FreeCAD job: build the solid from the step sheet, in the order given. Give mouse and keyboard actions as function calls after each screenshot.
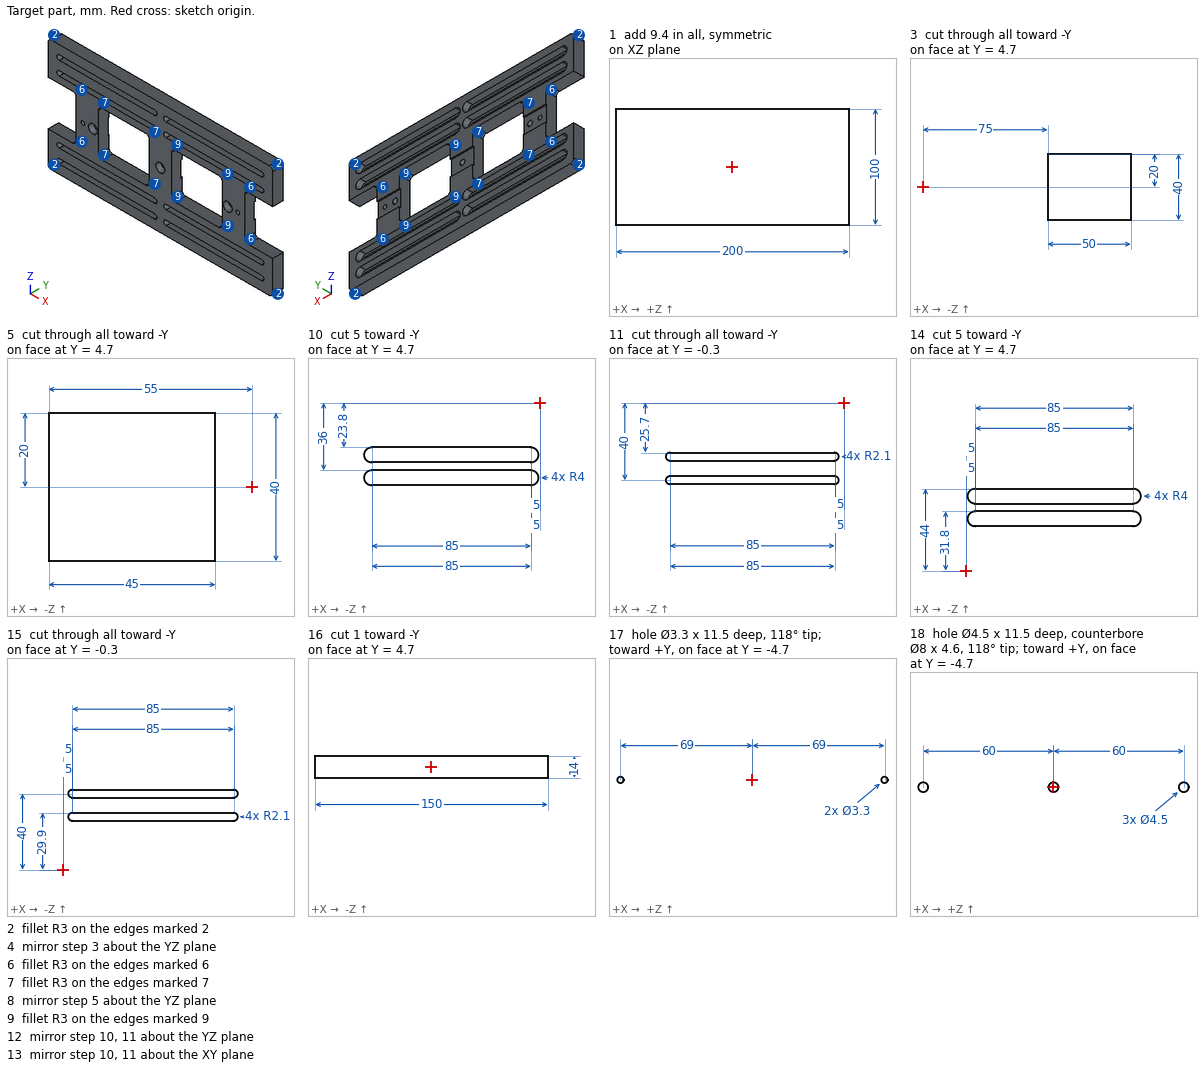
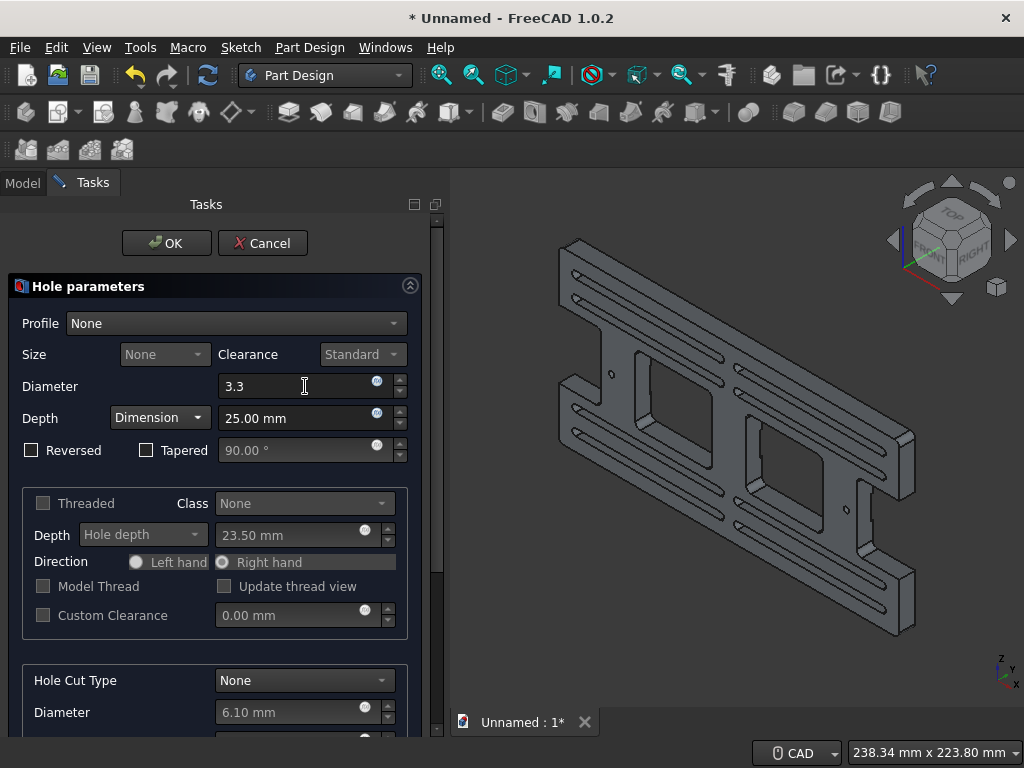
triple_click(305, 418)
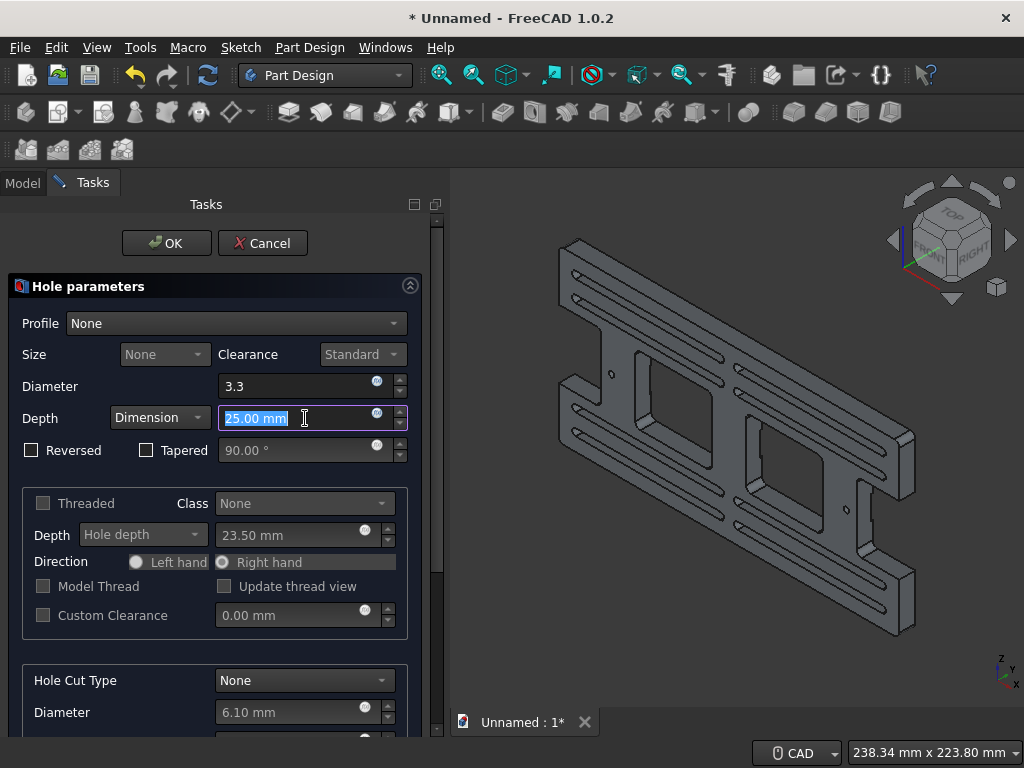
text(11.5)
key(Tab)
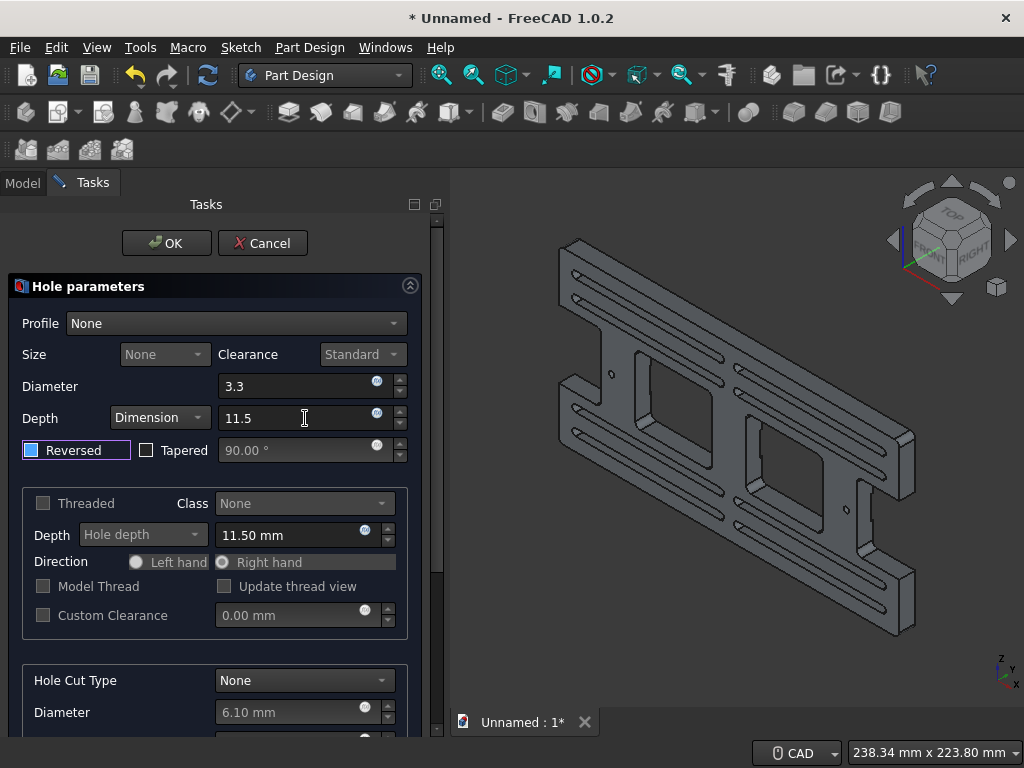
click(167, 243)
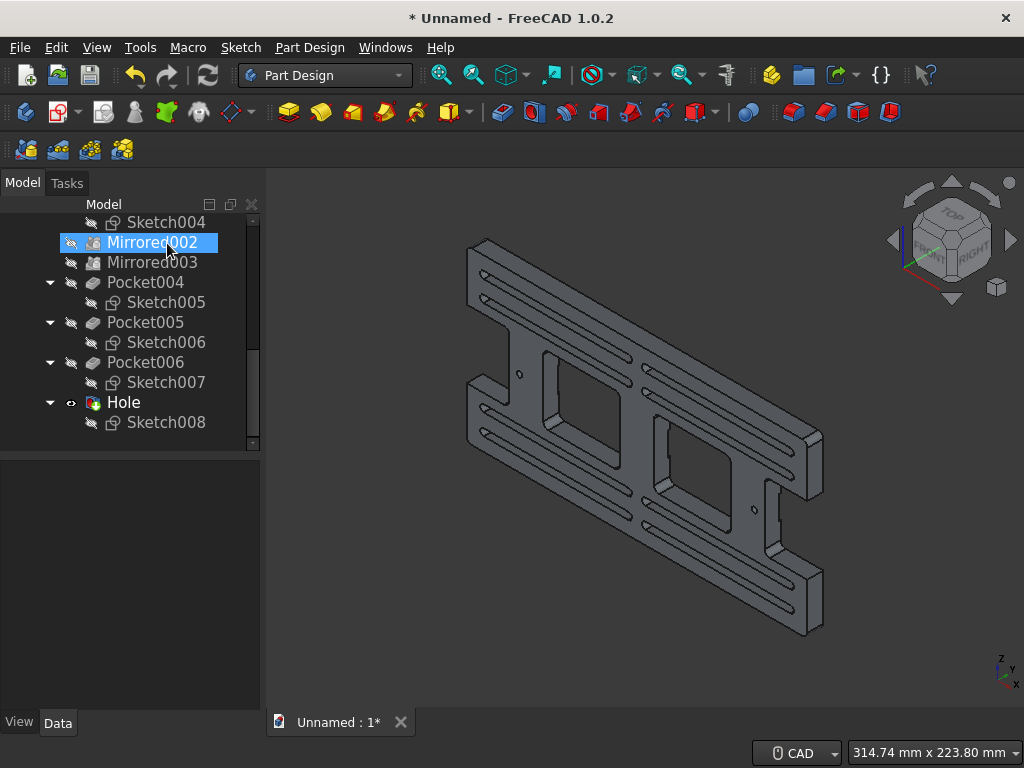
click(637, 469)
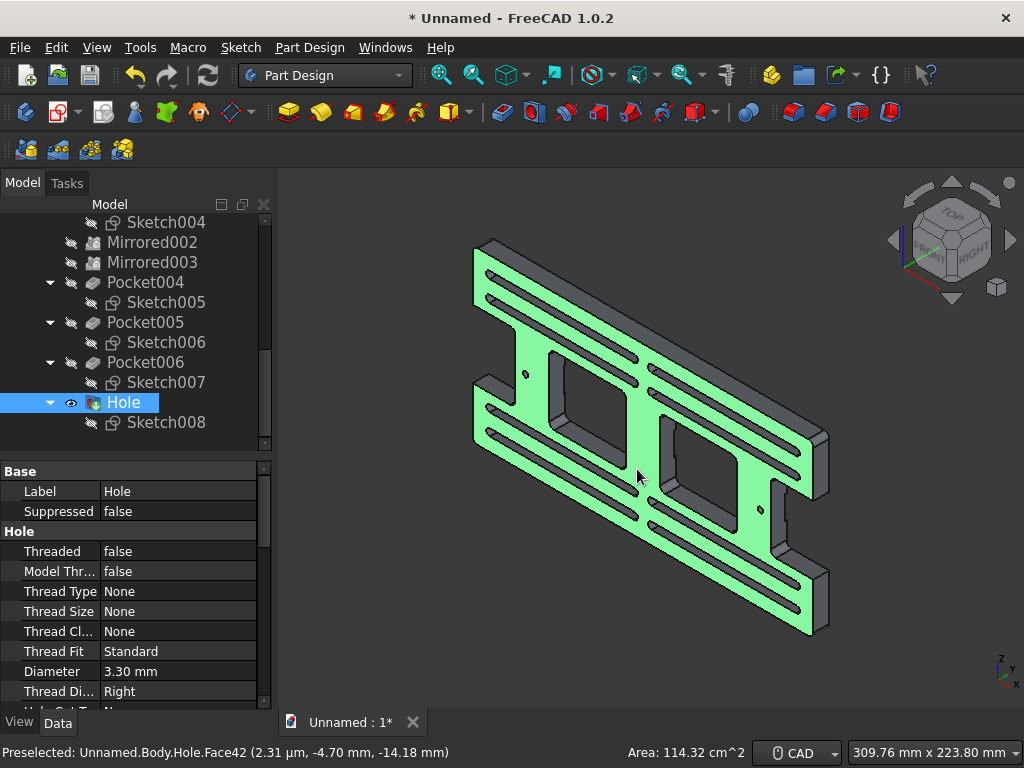
click(58, 112)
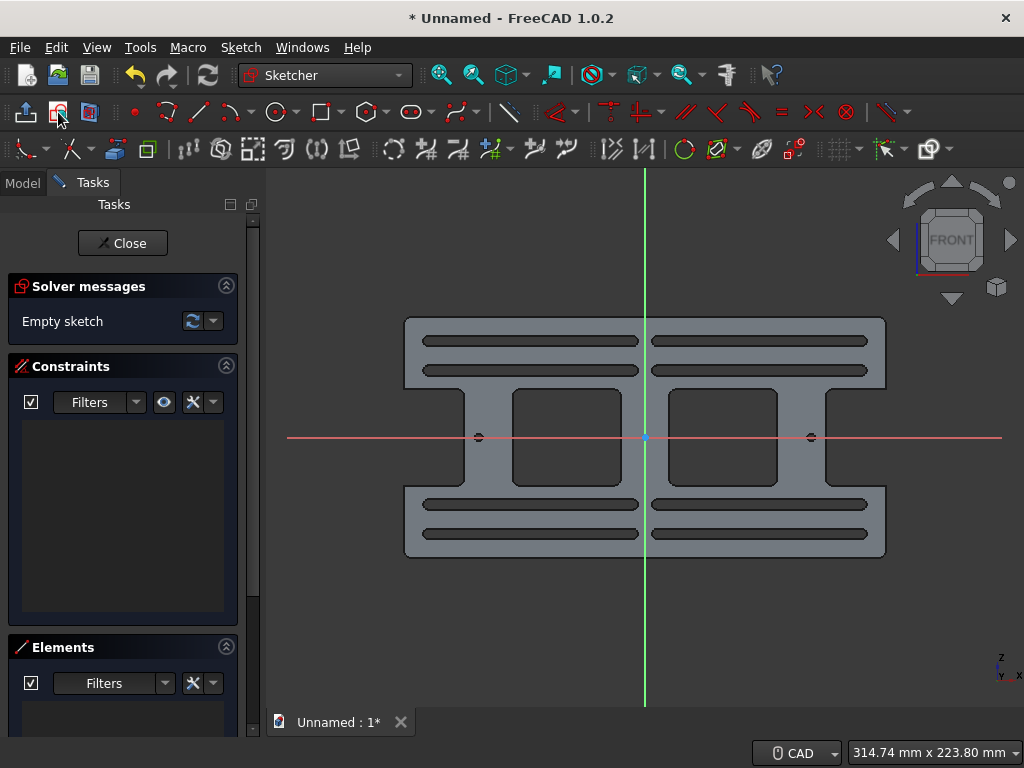
key(g)
key(c)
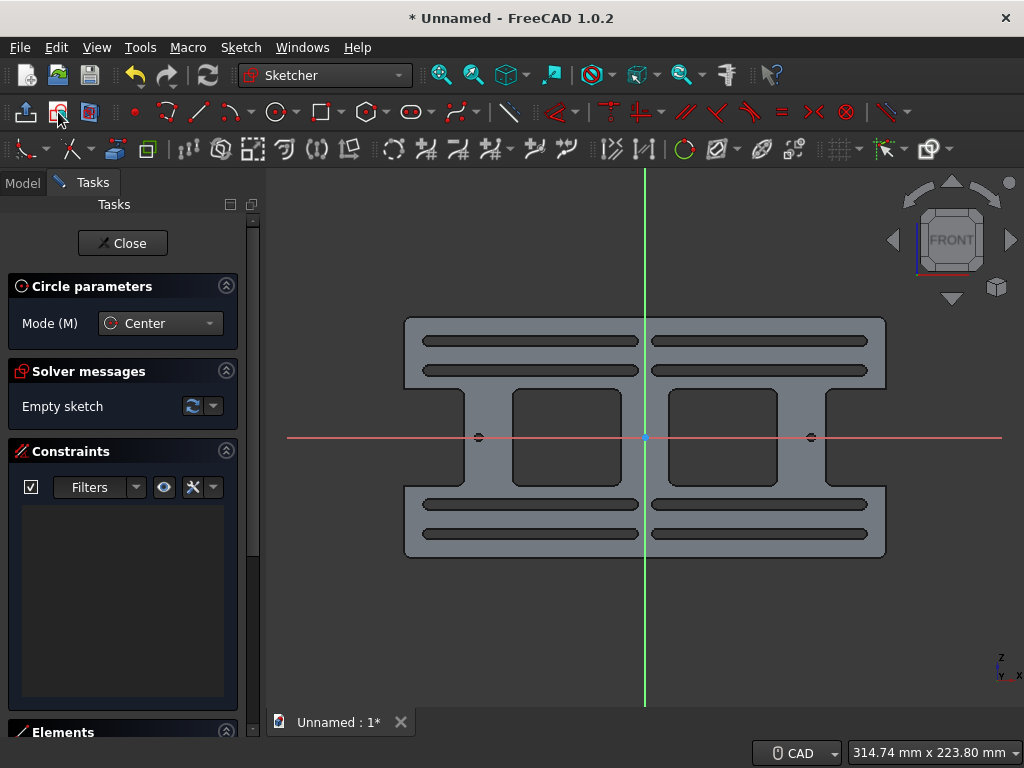
scroll(790, 438, up, 8)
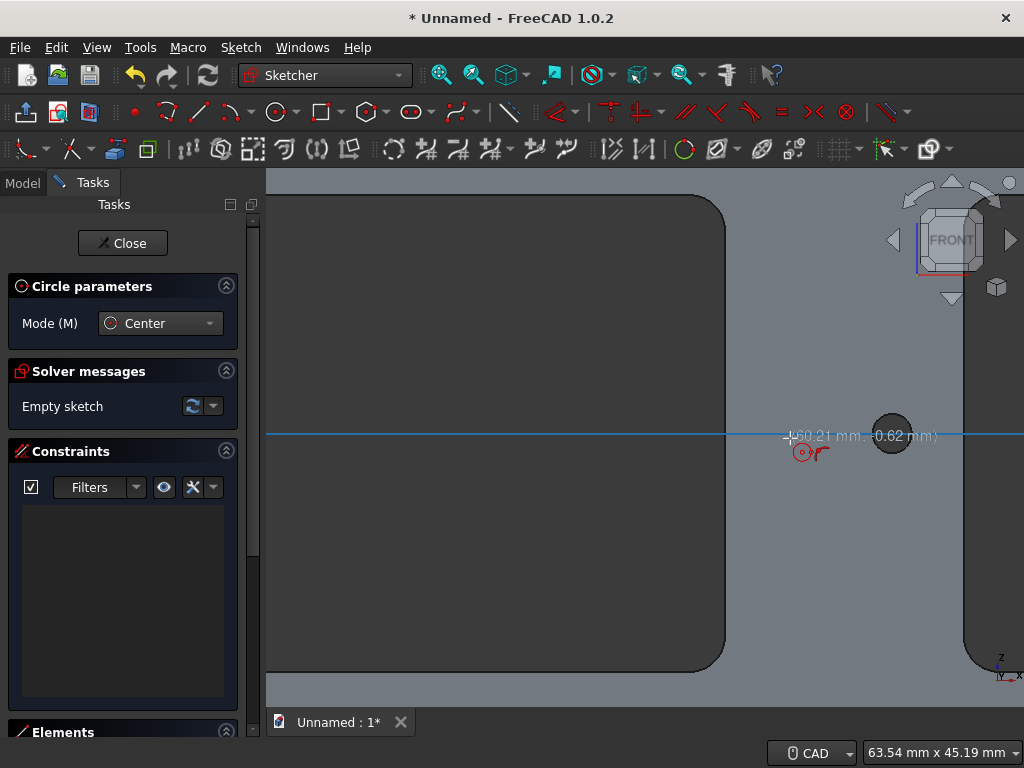
scroll(743, 439, down, 7)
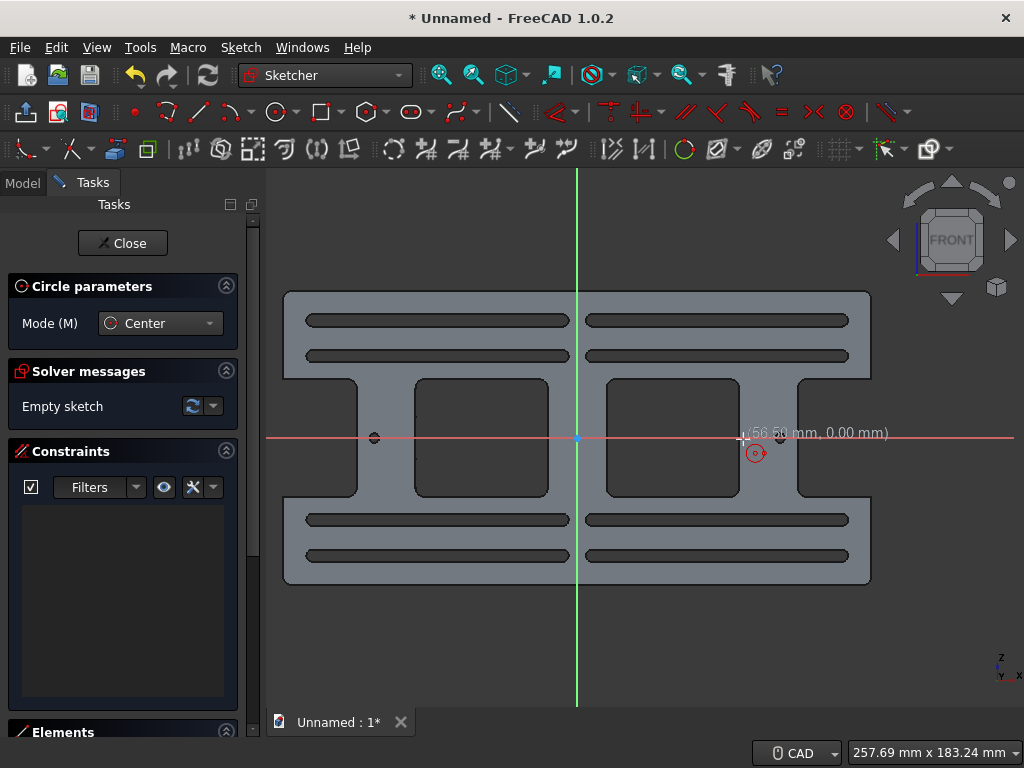
click(754, 438)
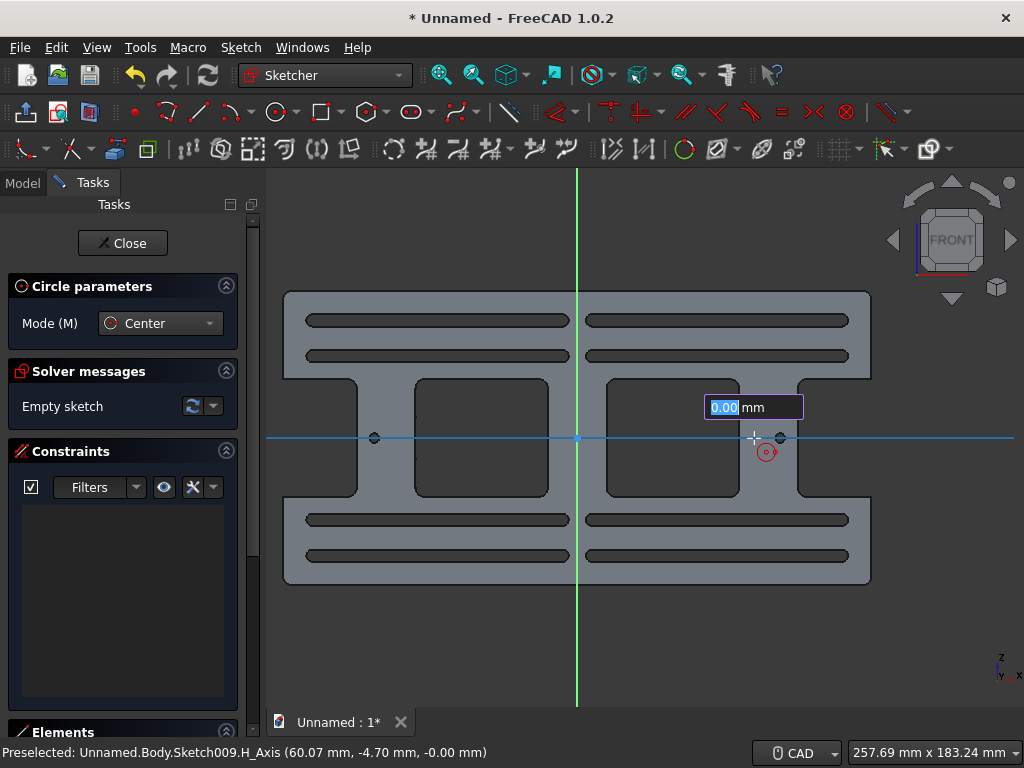
scroll(752, 444, up, 5)
move(750, 444)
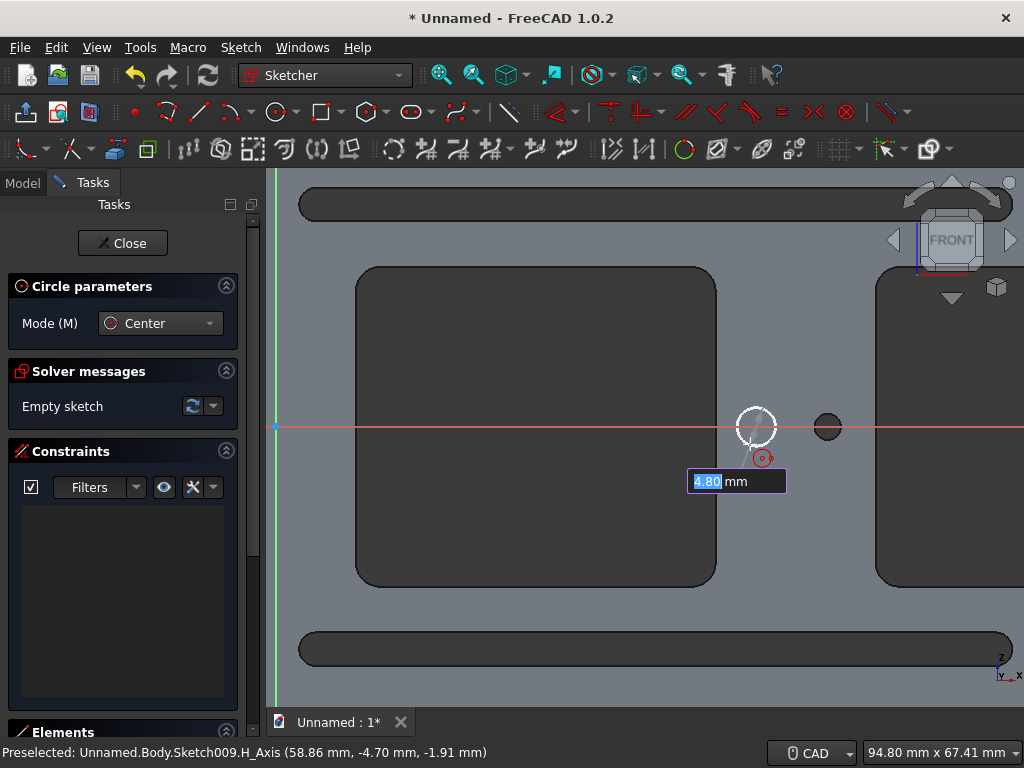
text(4.5)
key(Return)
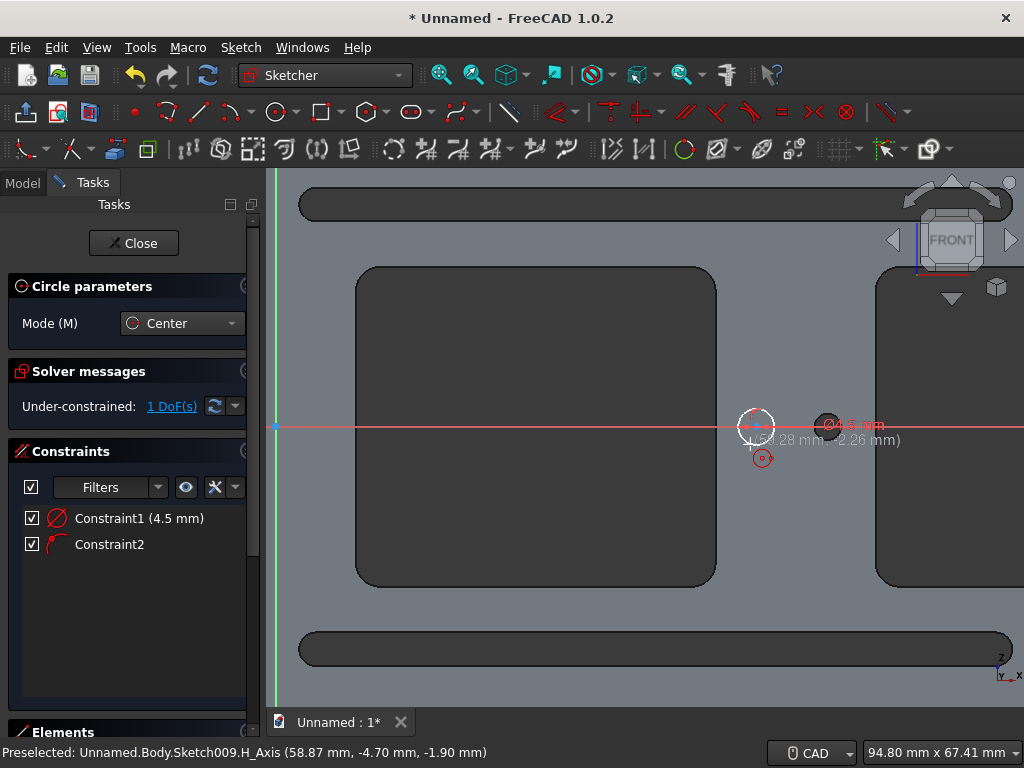
scroll(751, 444, down, 5)